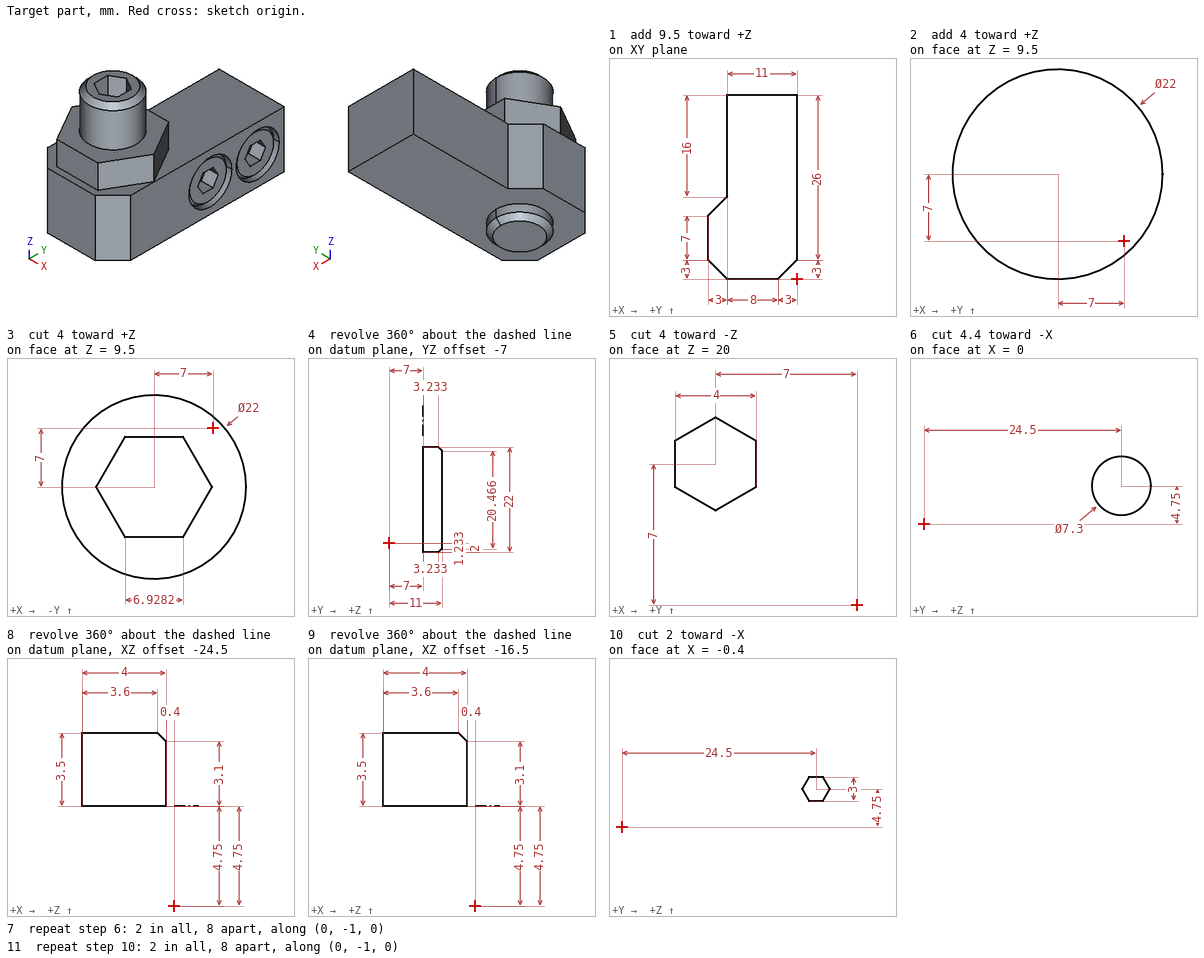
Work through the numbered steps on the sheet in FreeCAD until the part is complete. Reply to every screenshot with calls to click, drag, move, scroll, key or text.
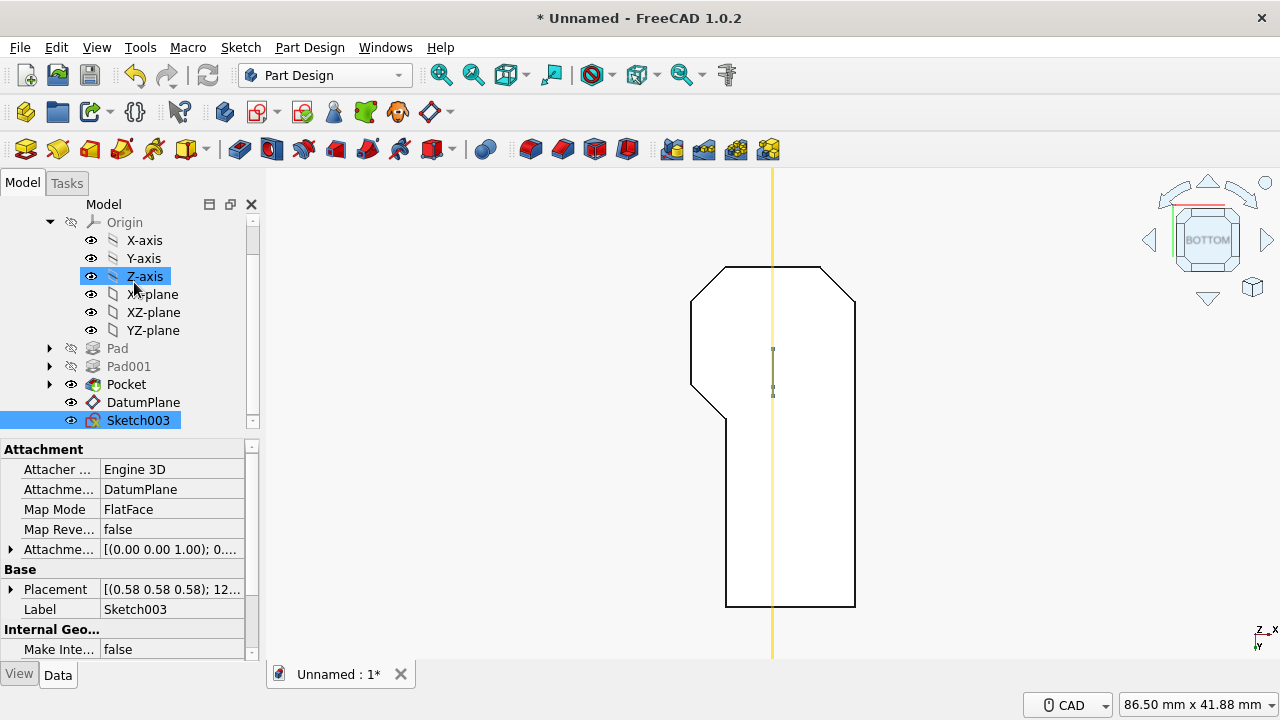
click(58, 150)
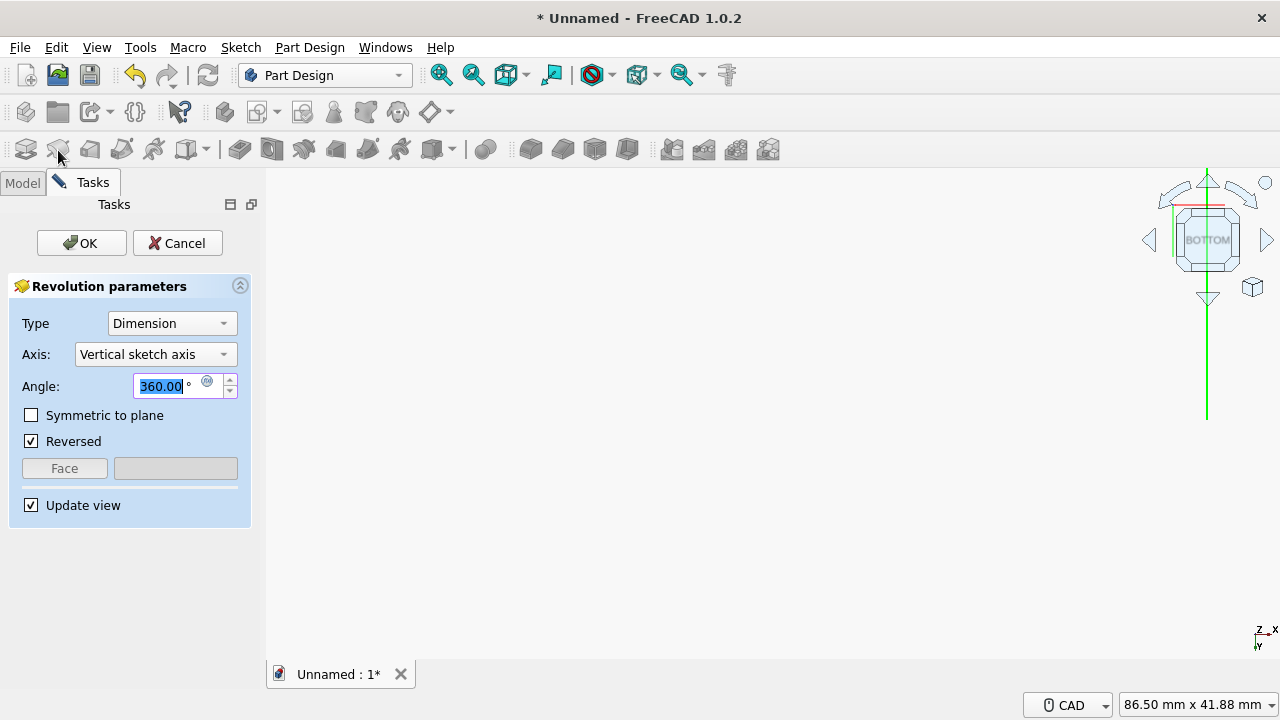
click(156, 354)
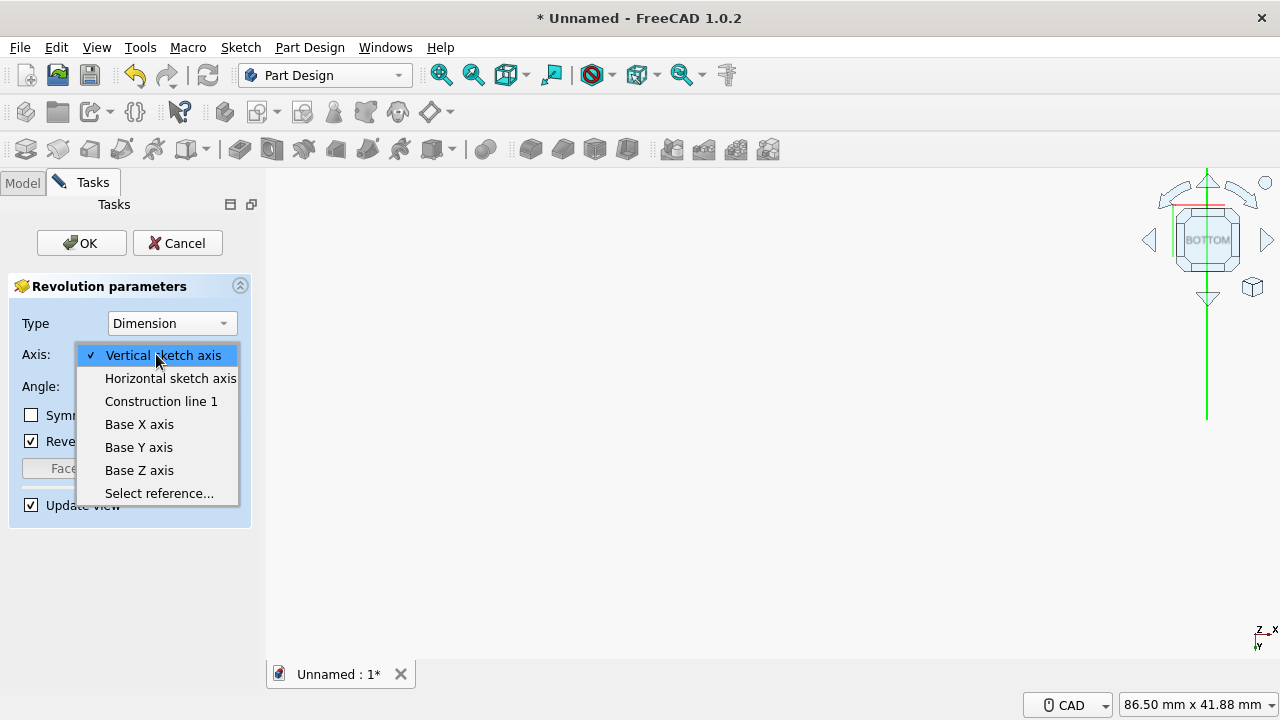
click(156, 402)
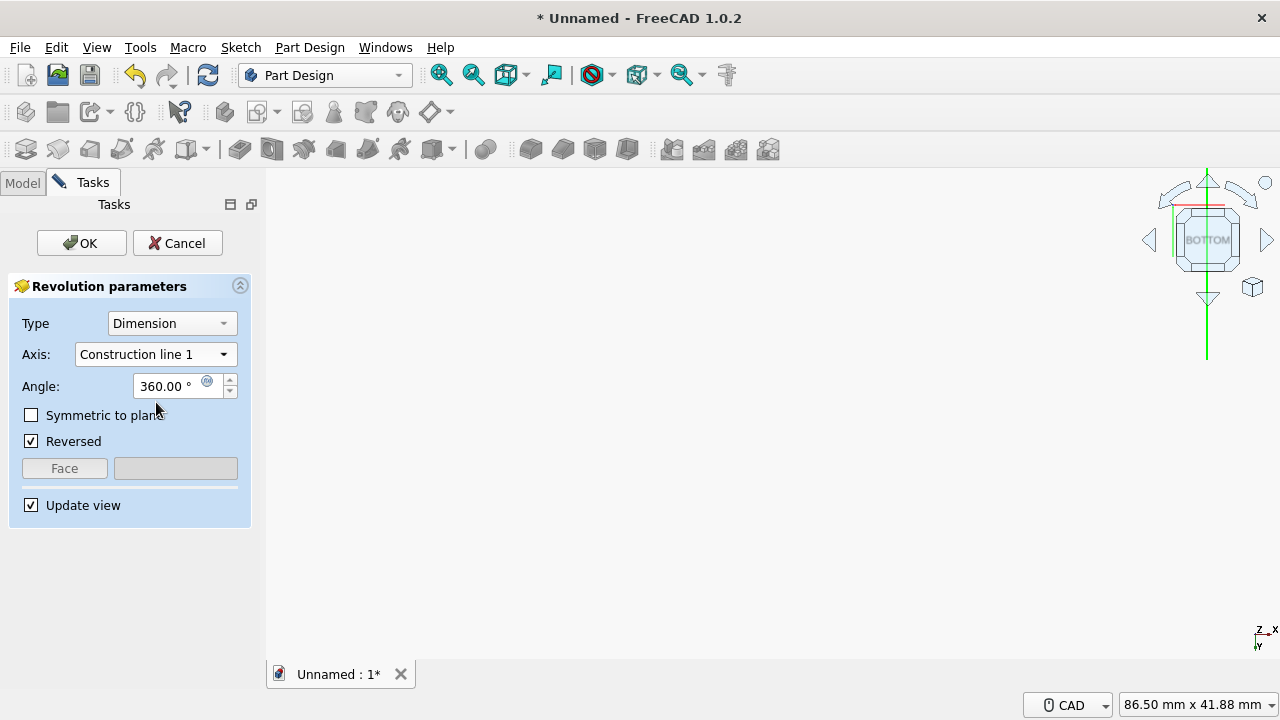
click(82, 243)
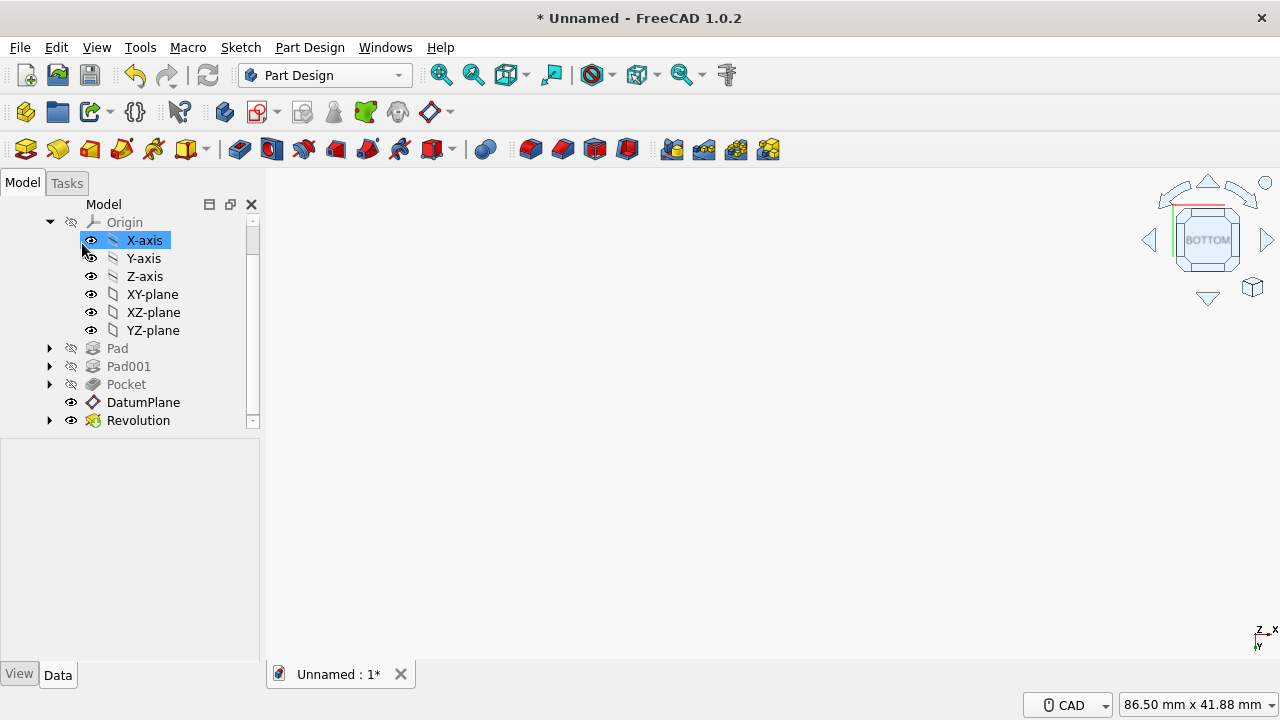
click(116, 402)
key(space)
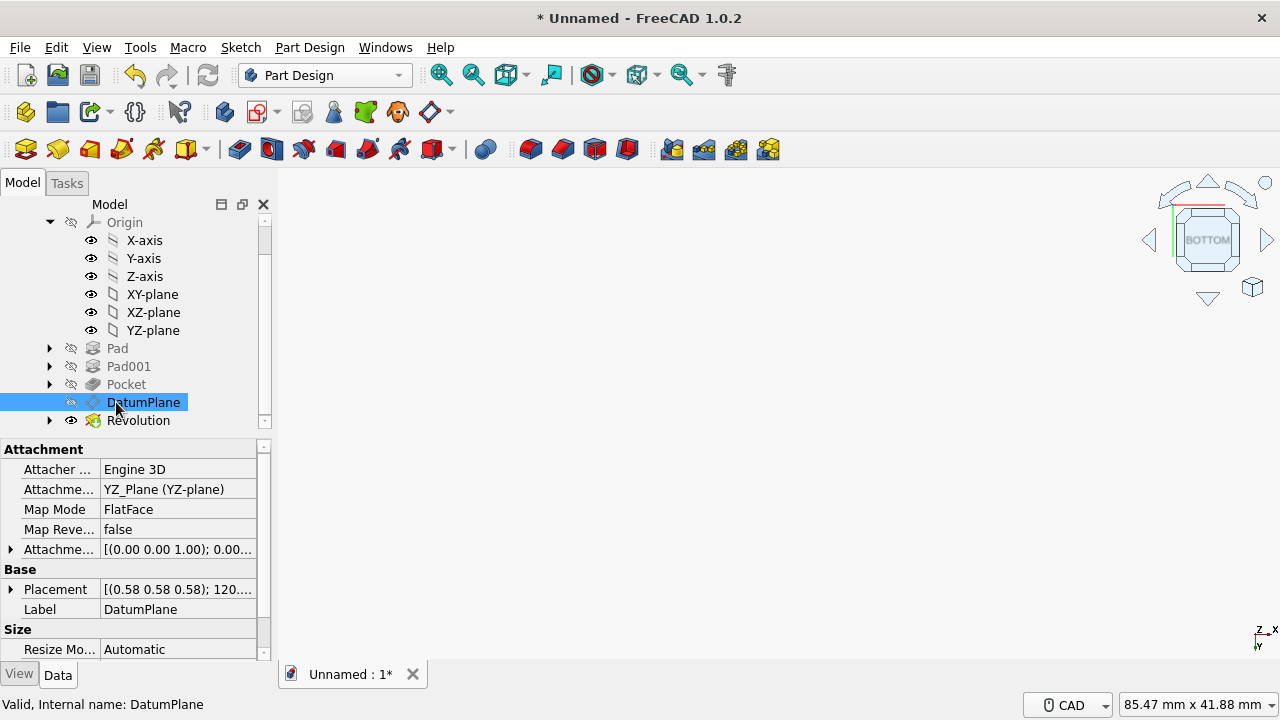
key(v)
key(f)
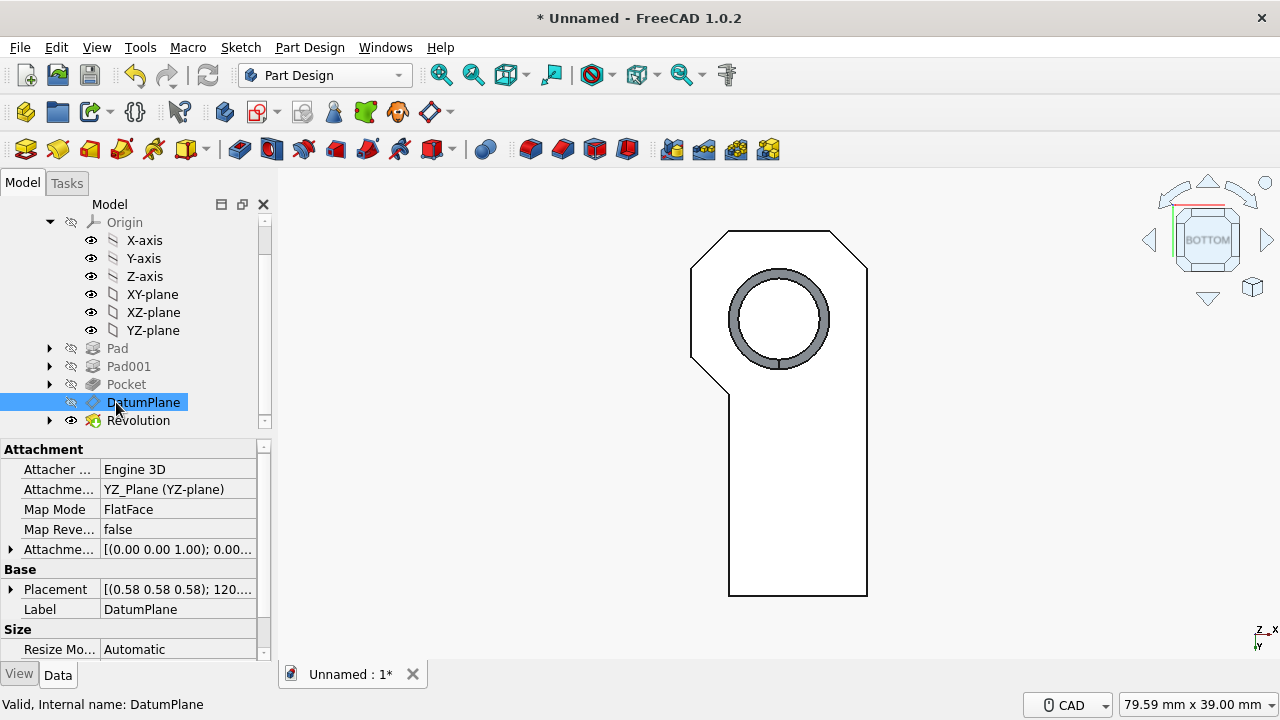
key(0)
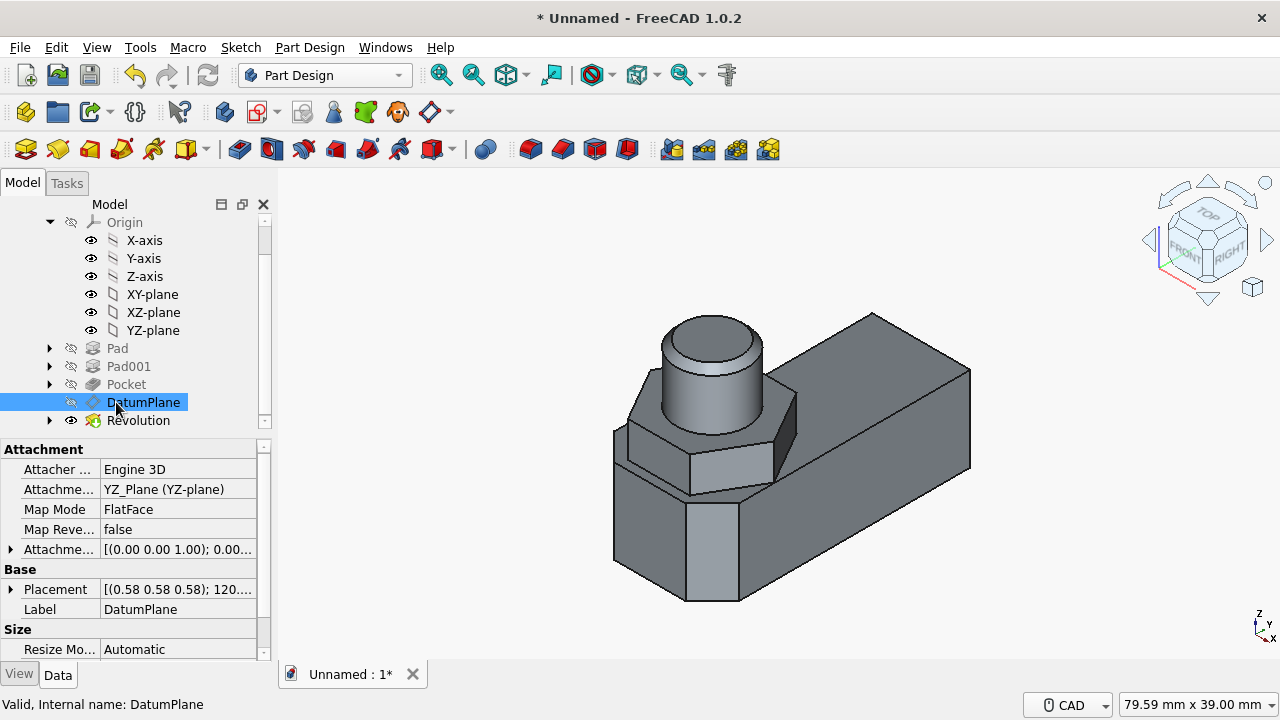
click(712, 338)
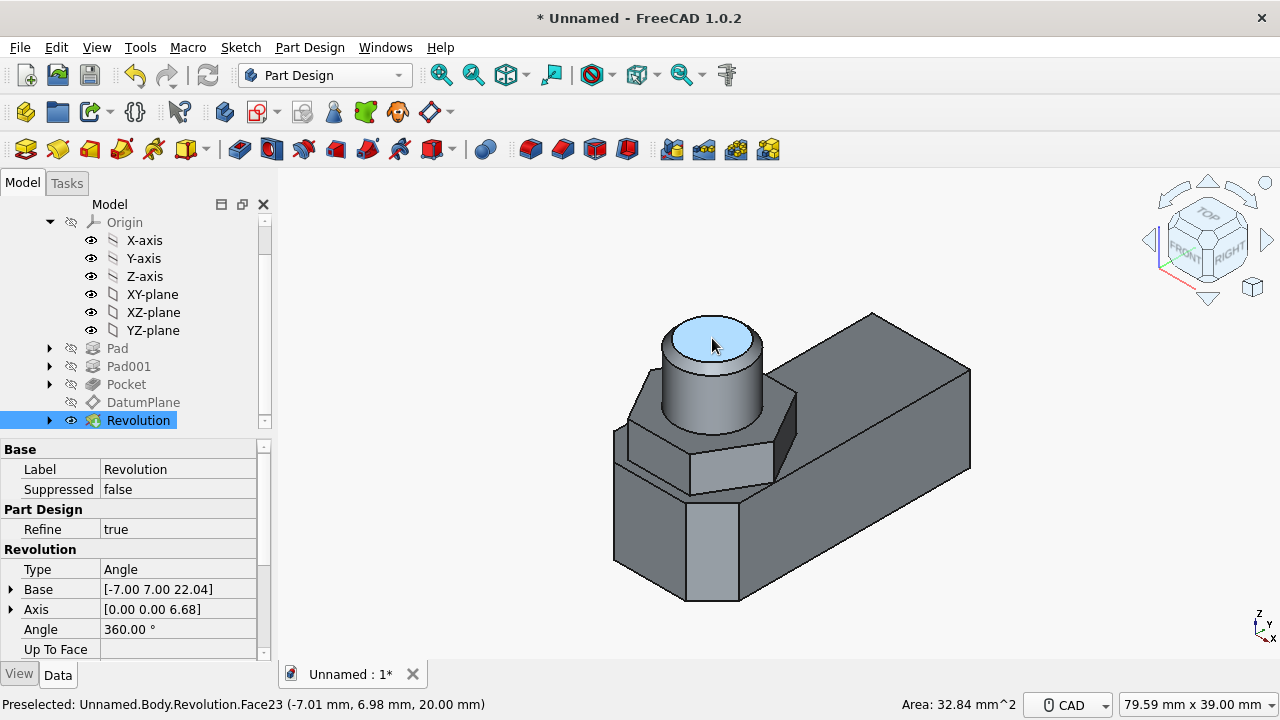
click(258, 112)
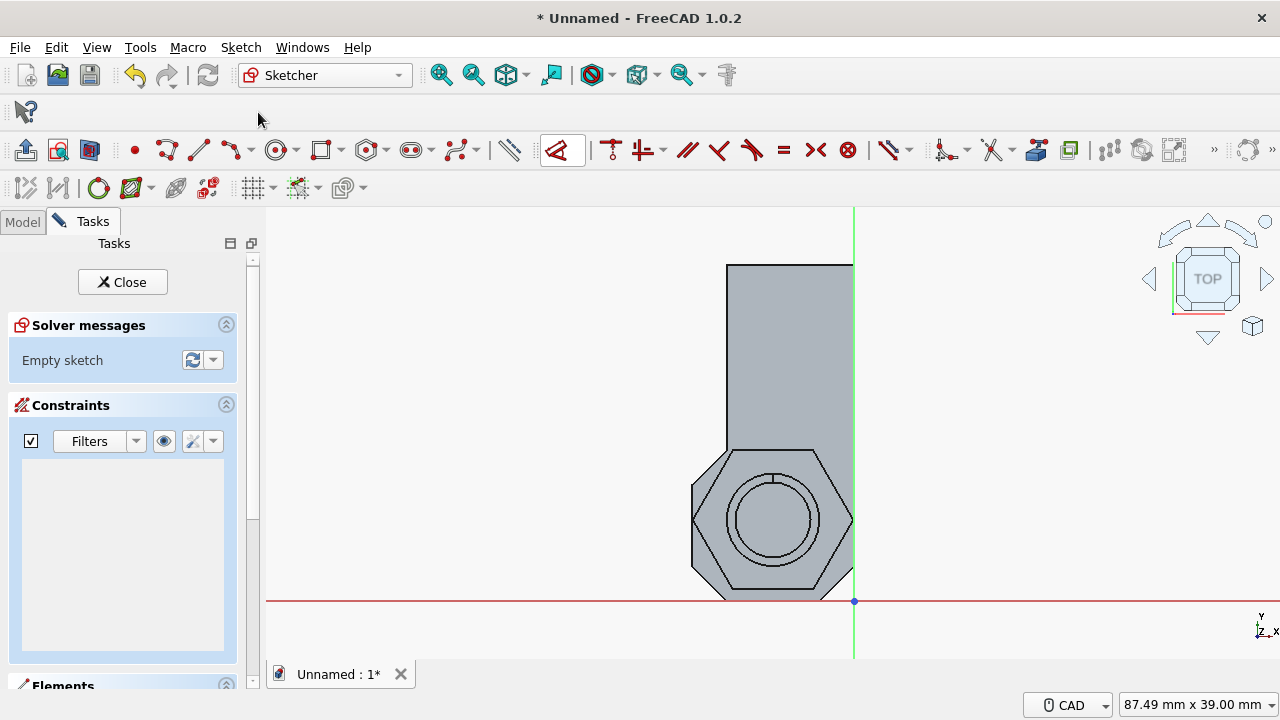
scroll(859, 614, up, 5)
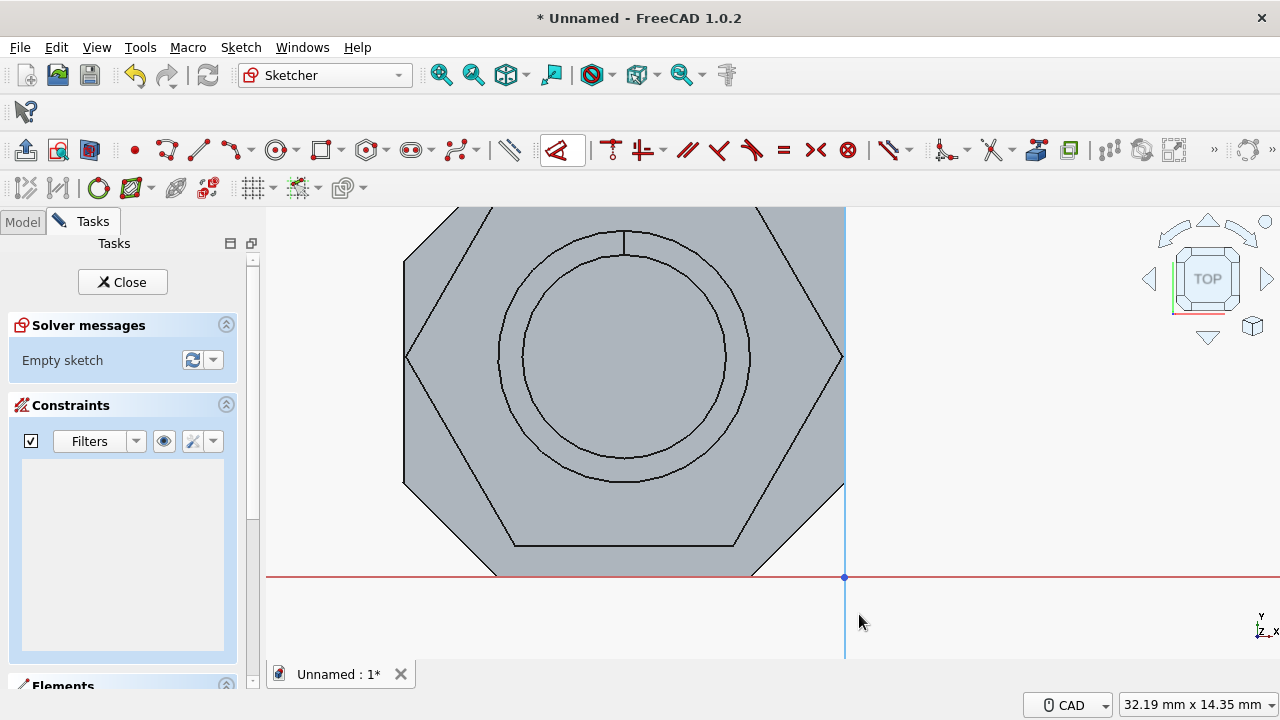
click(366, 150)